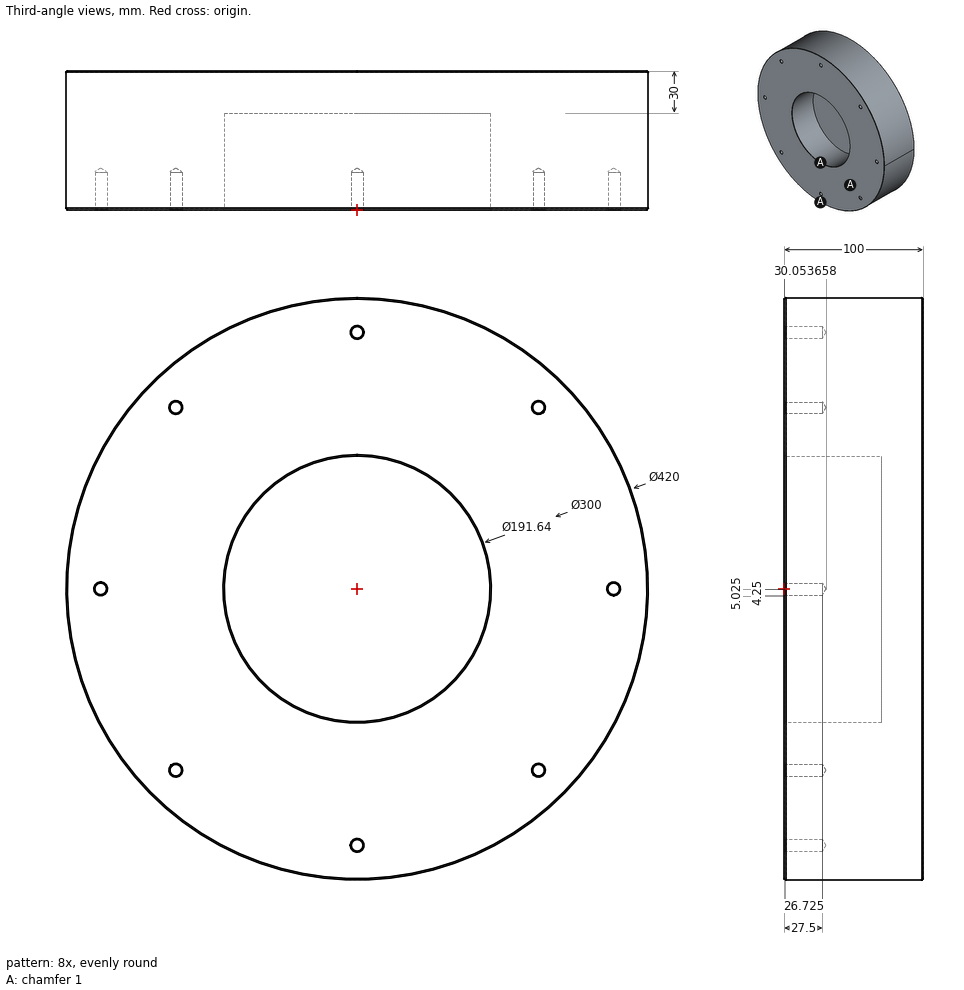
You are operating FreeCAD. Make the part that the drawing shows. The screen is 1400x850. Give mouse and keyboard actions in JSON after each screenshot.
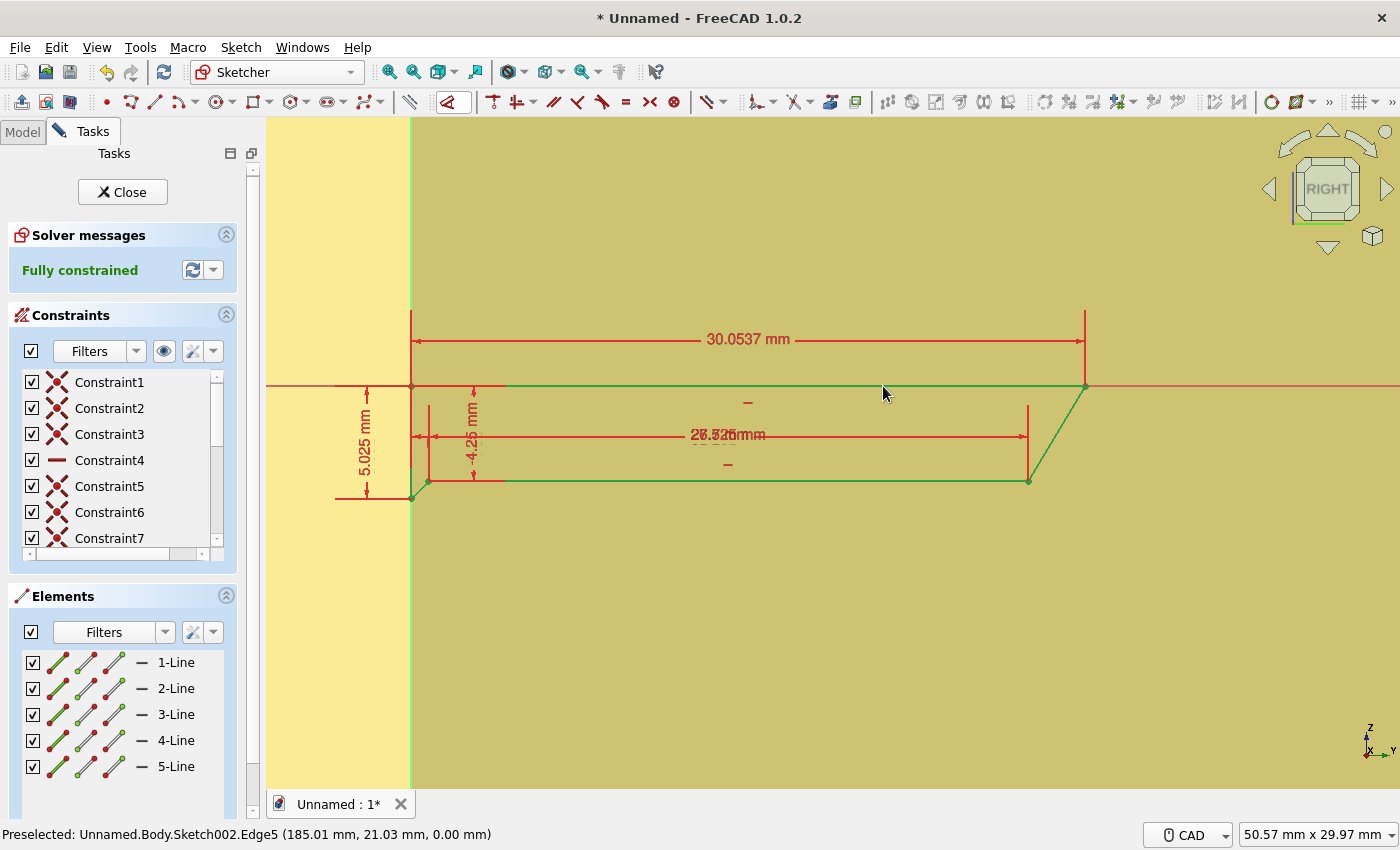
{"action": "left_click", "coordinate": [123, 192]}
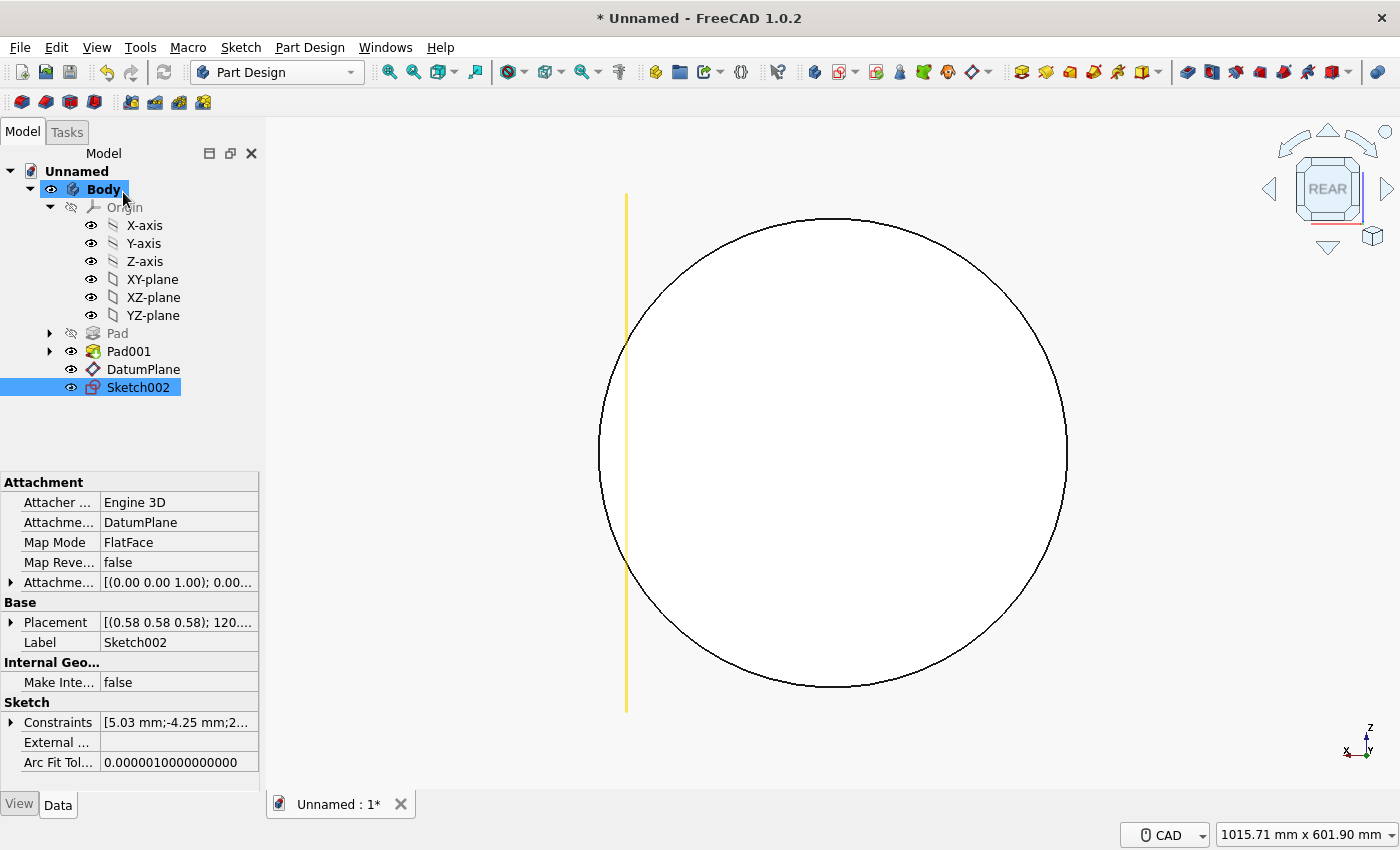
{"action": "left_click", "coordinate": [1236, 72]}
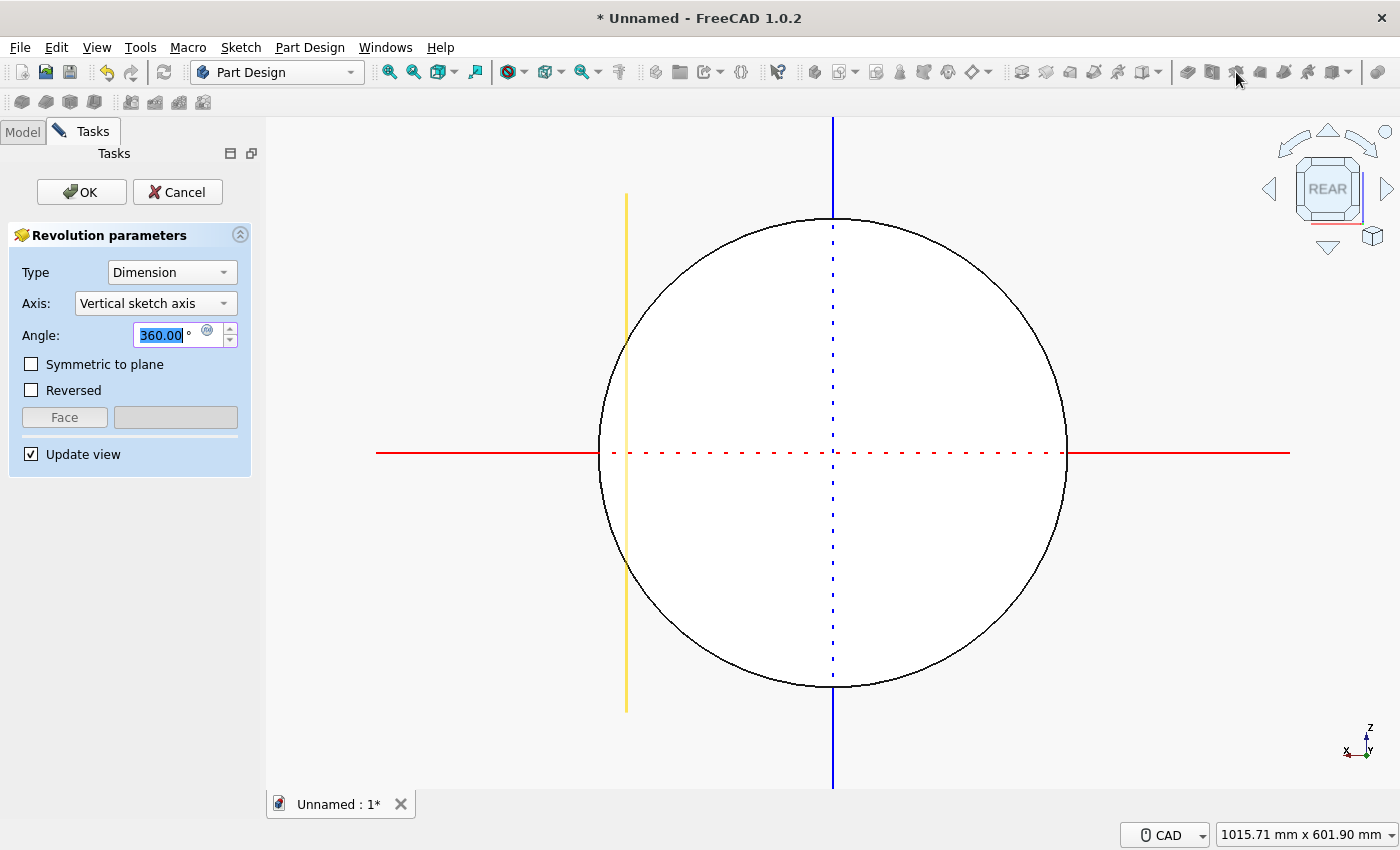
{"action": "left_click", "coordinate": [156, 304]}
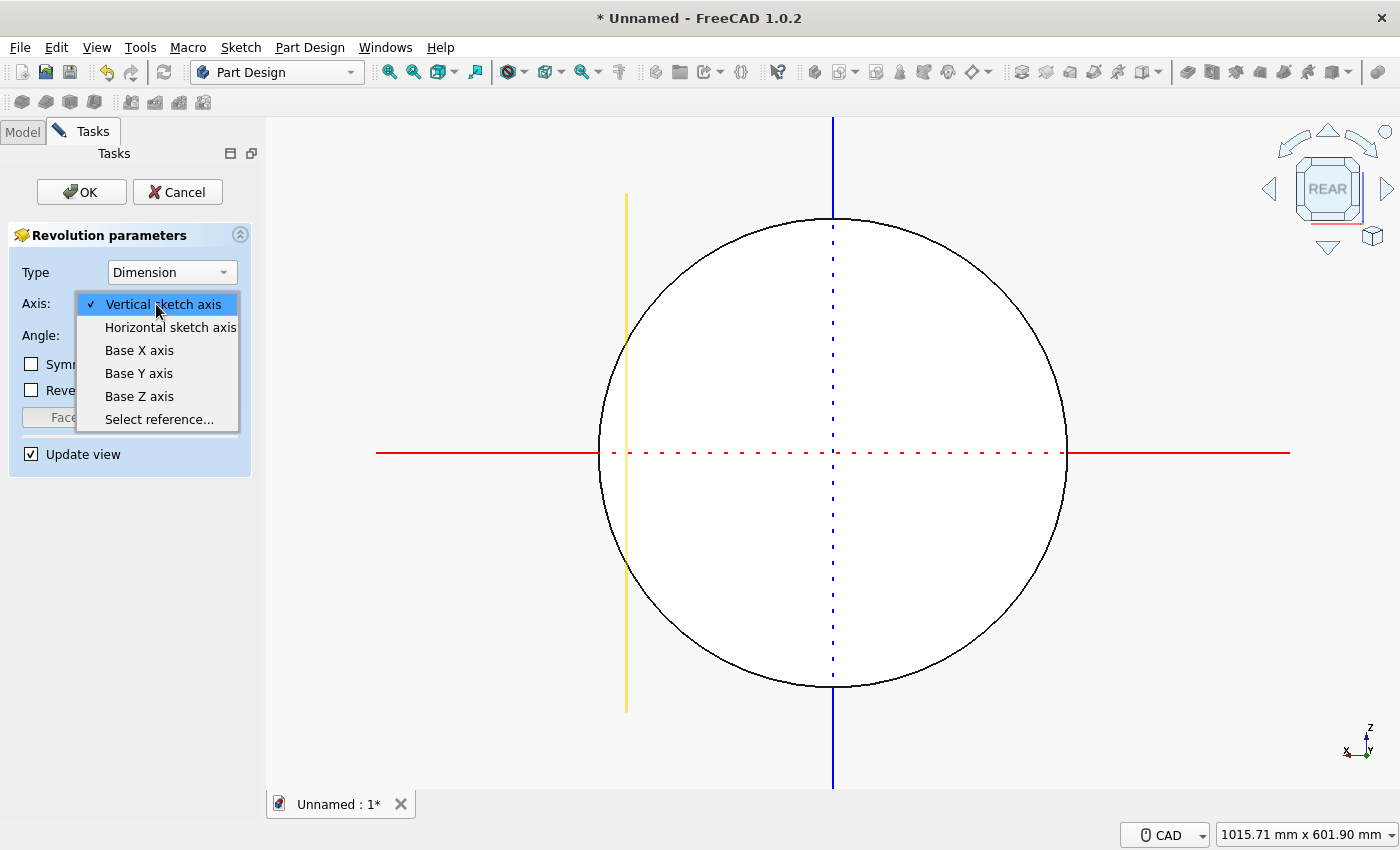
{"action": "left_click", "coordinate": [156, 328]}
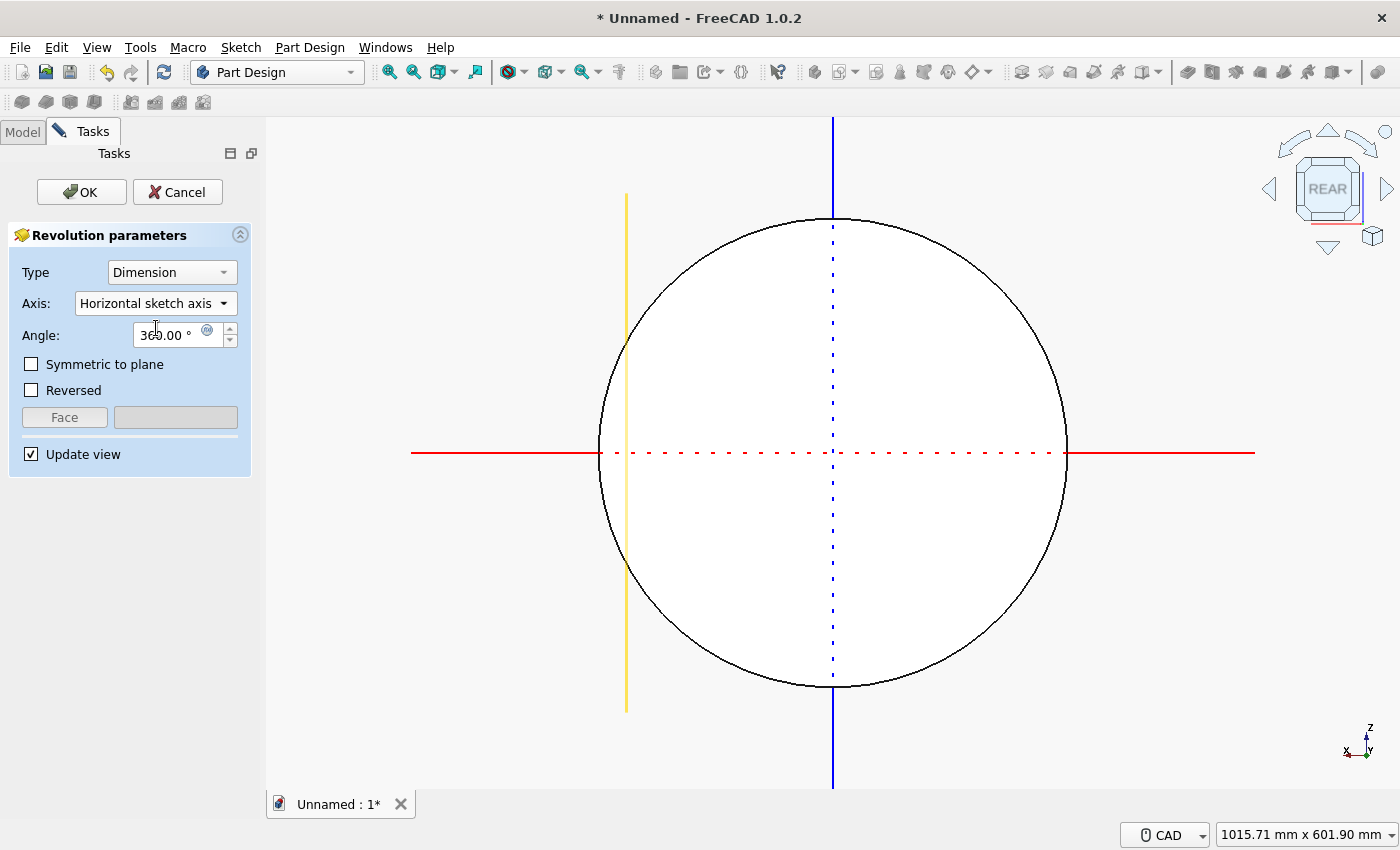
{"action": "left_click", "coordinate": [82, 192]}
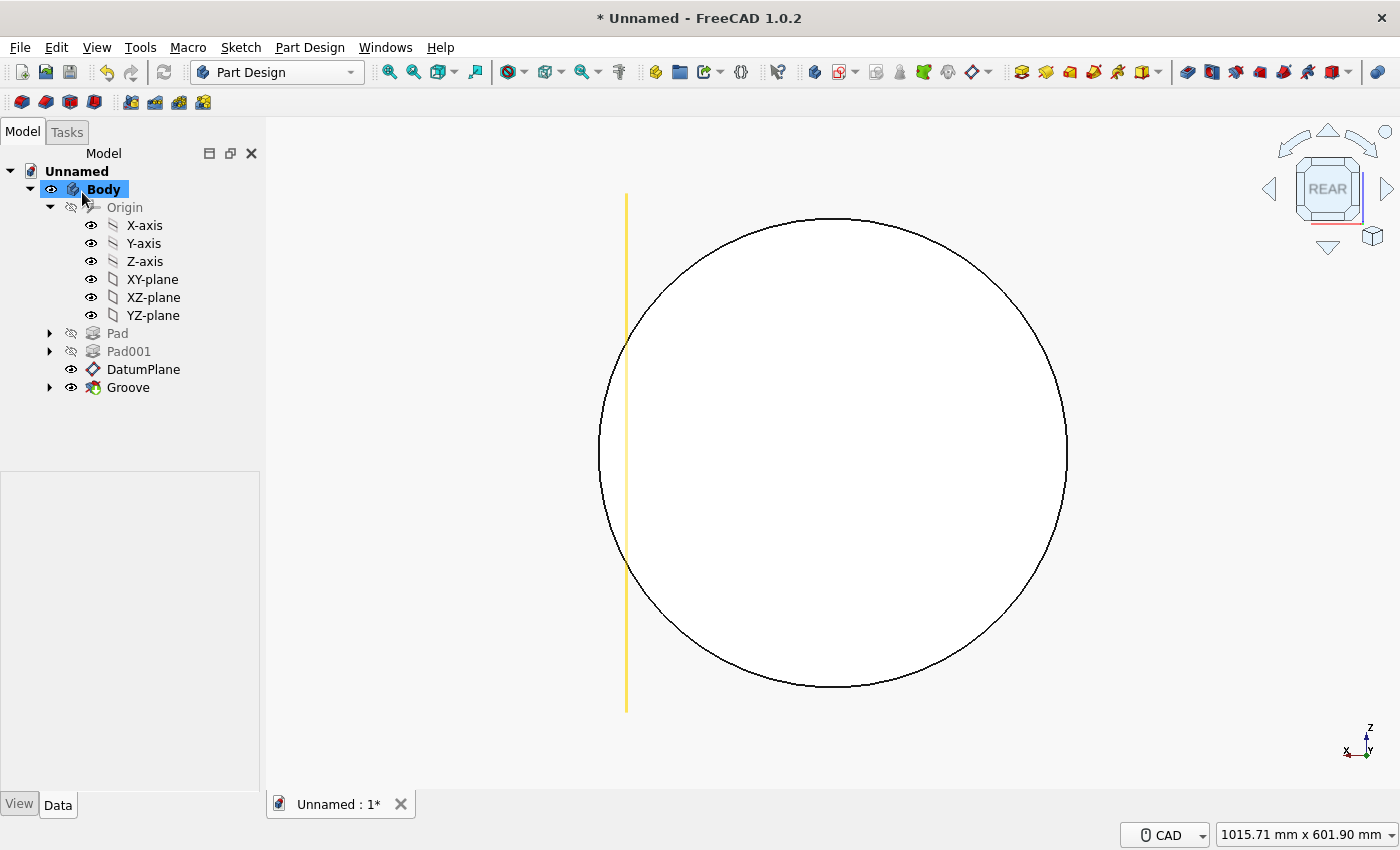
{"action": "left_click", "coordinate": [116, 369]}
{"action": "key", "text": "space"}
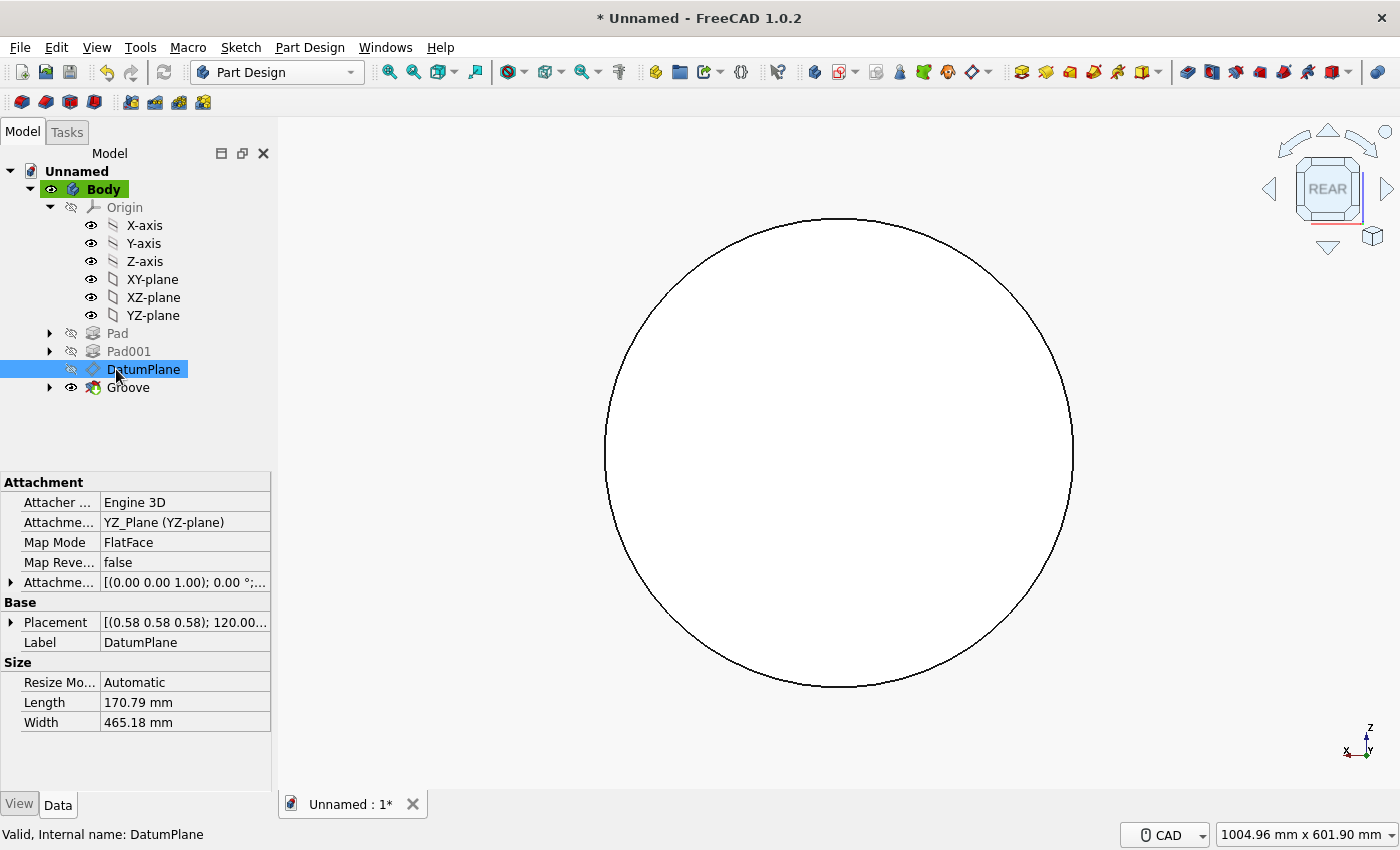
{"action": "left_click", "coordinate": [116, 387]}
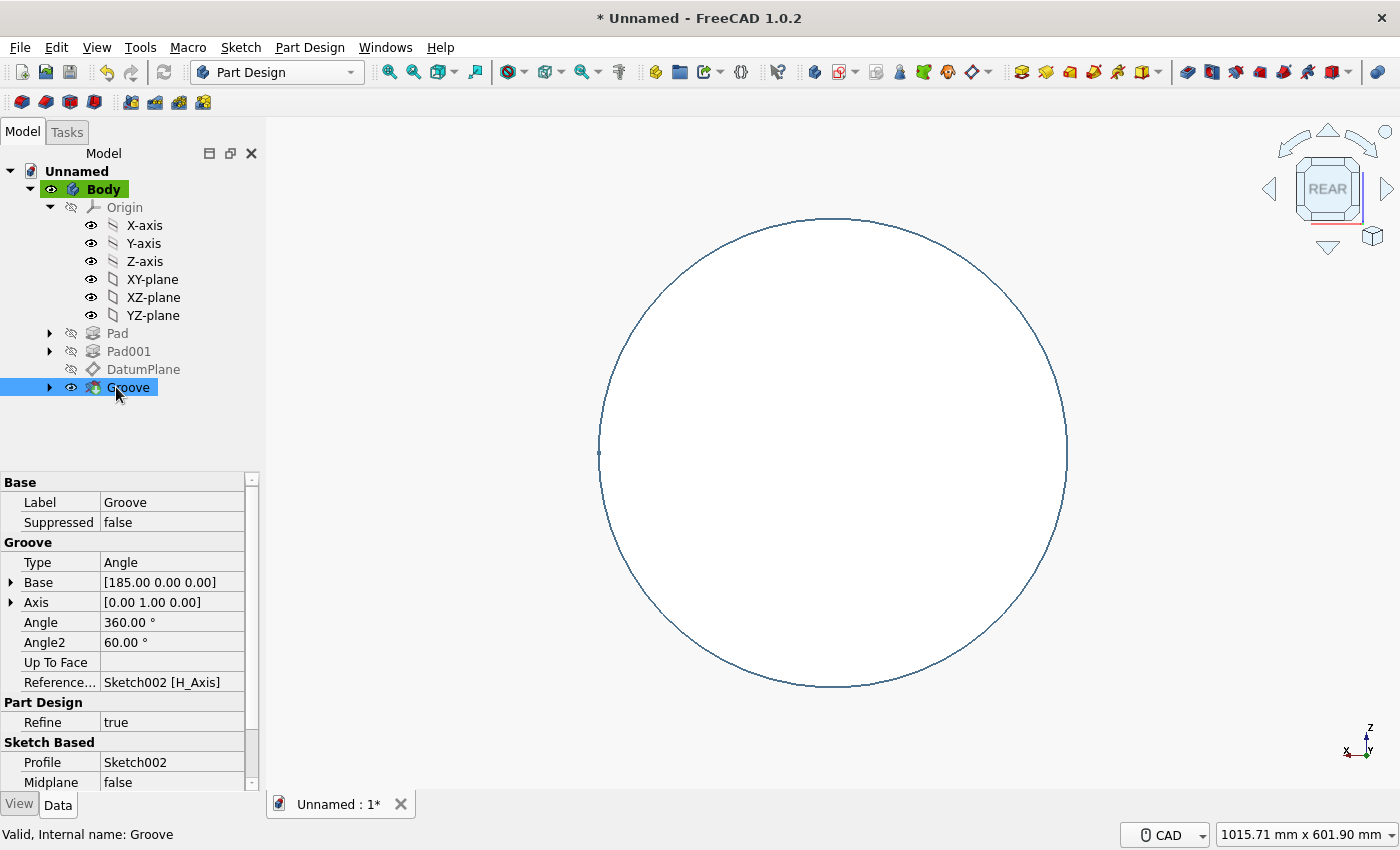
{"action": "left_click", "coordinate": [180, 102]}